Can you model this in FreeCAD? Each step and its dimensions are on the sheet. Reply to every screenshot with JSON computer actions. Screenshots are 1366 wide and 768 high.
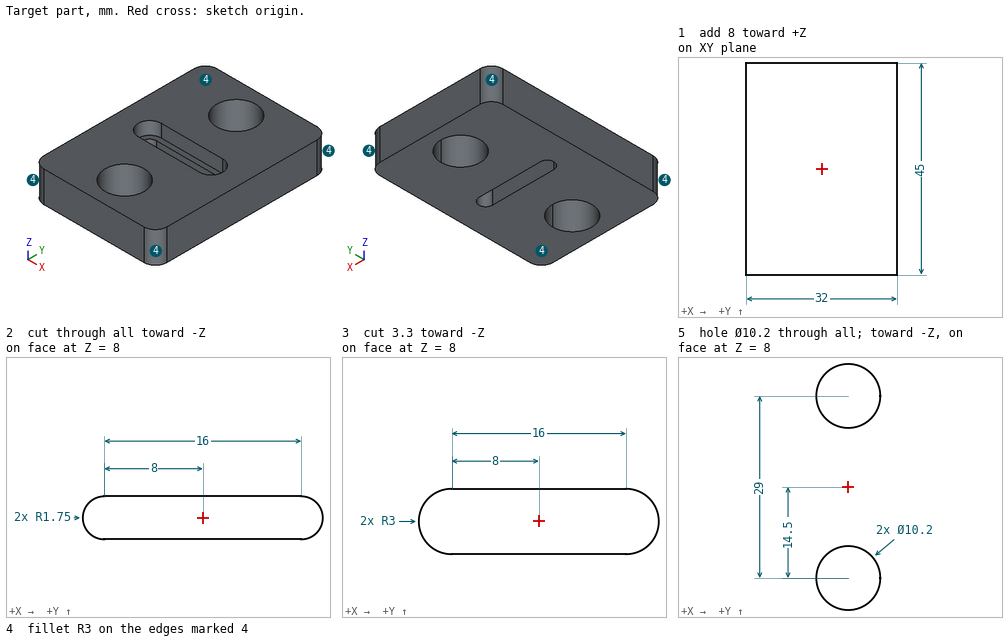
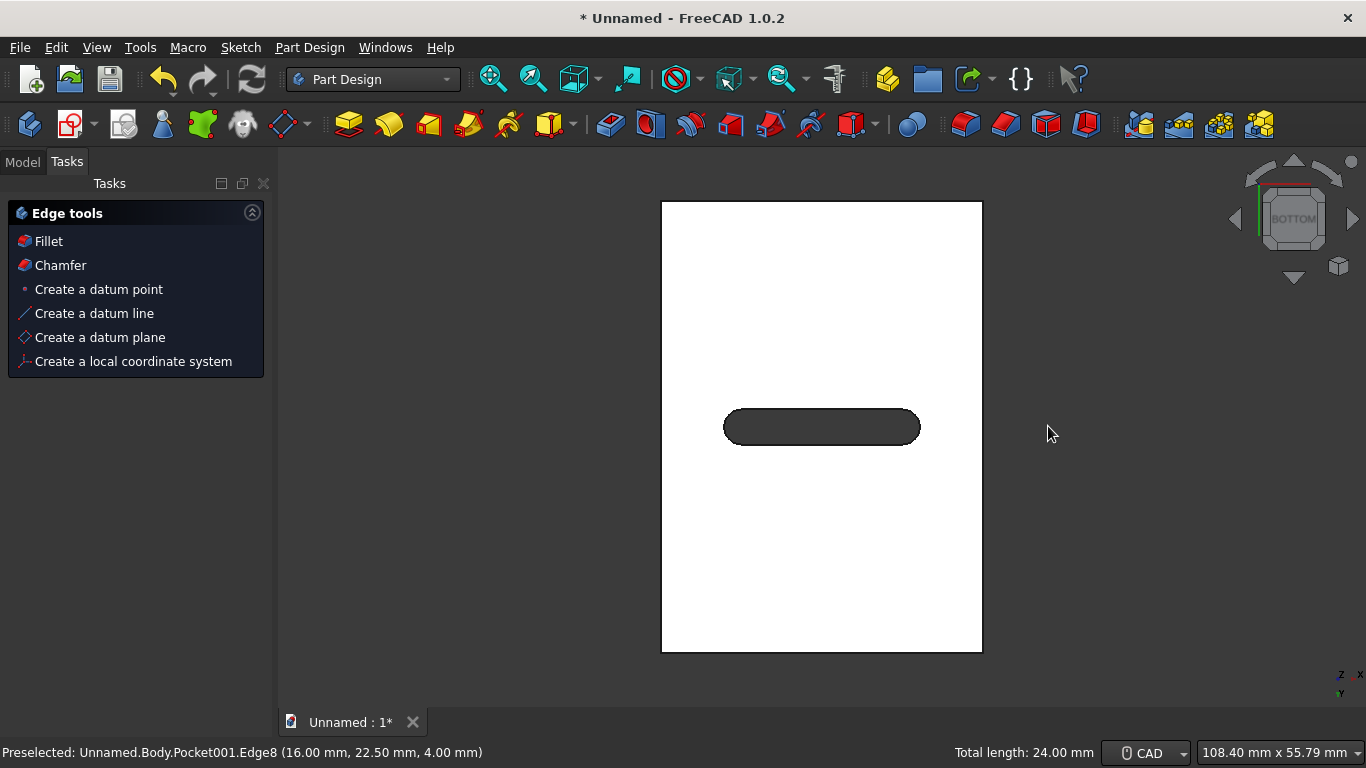
{"action": "key", "text": "4"}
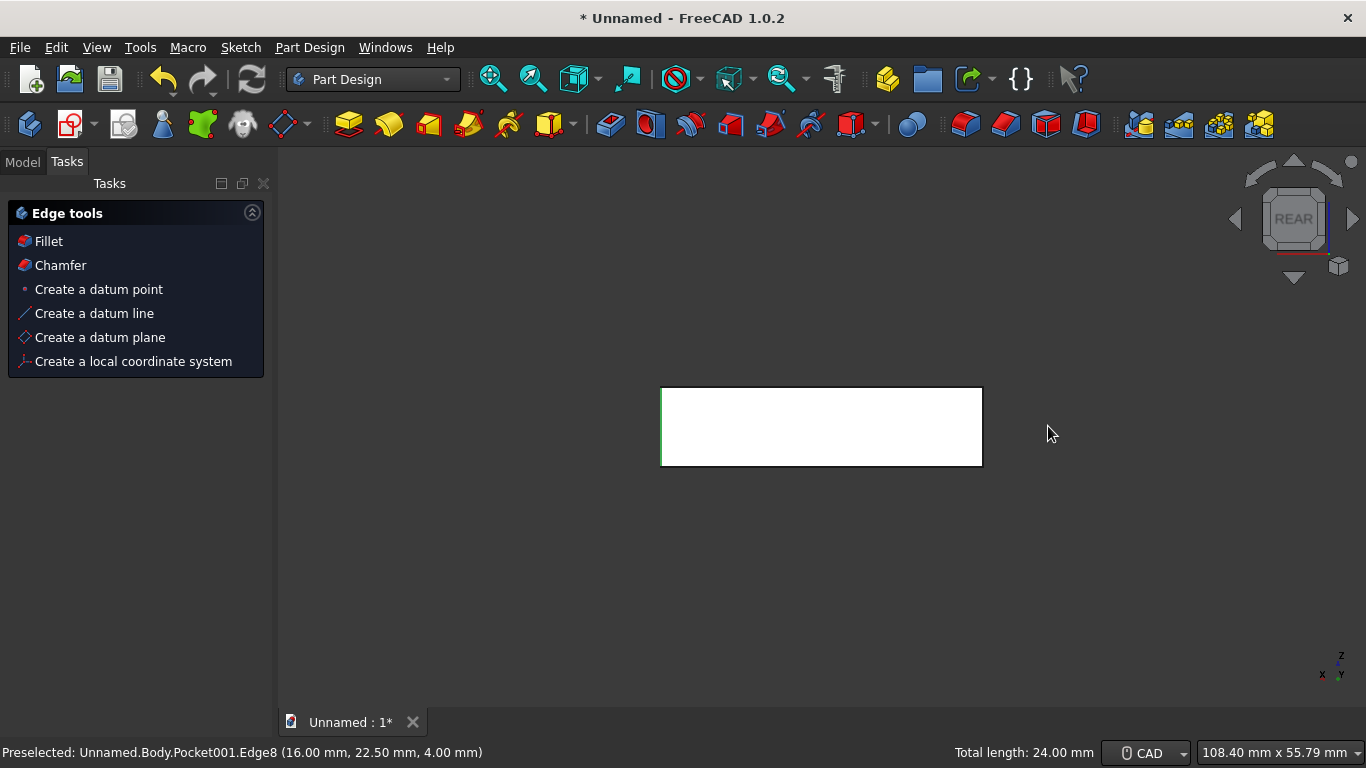
{"action": "key", "text": "v f"}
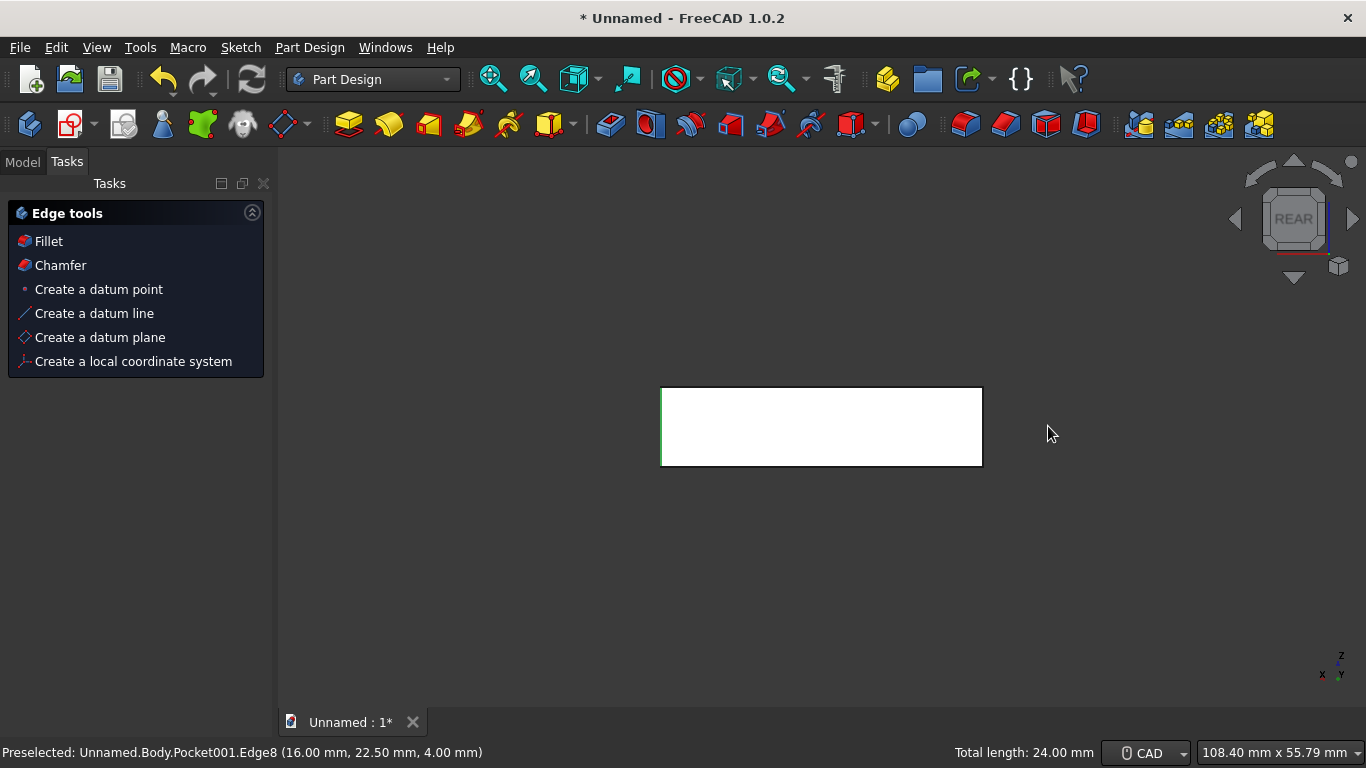
{"action": "left_click", "coordinate": [983, 426], "text": "ctrl"}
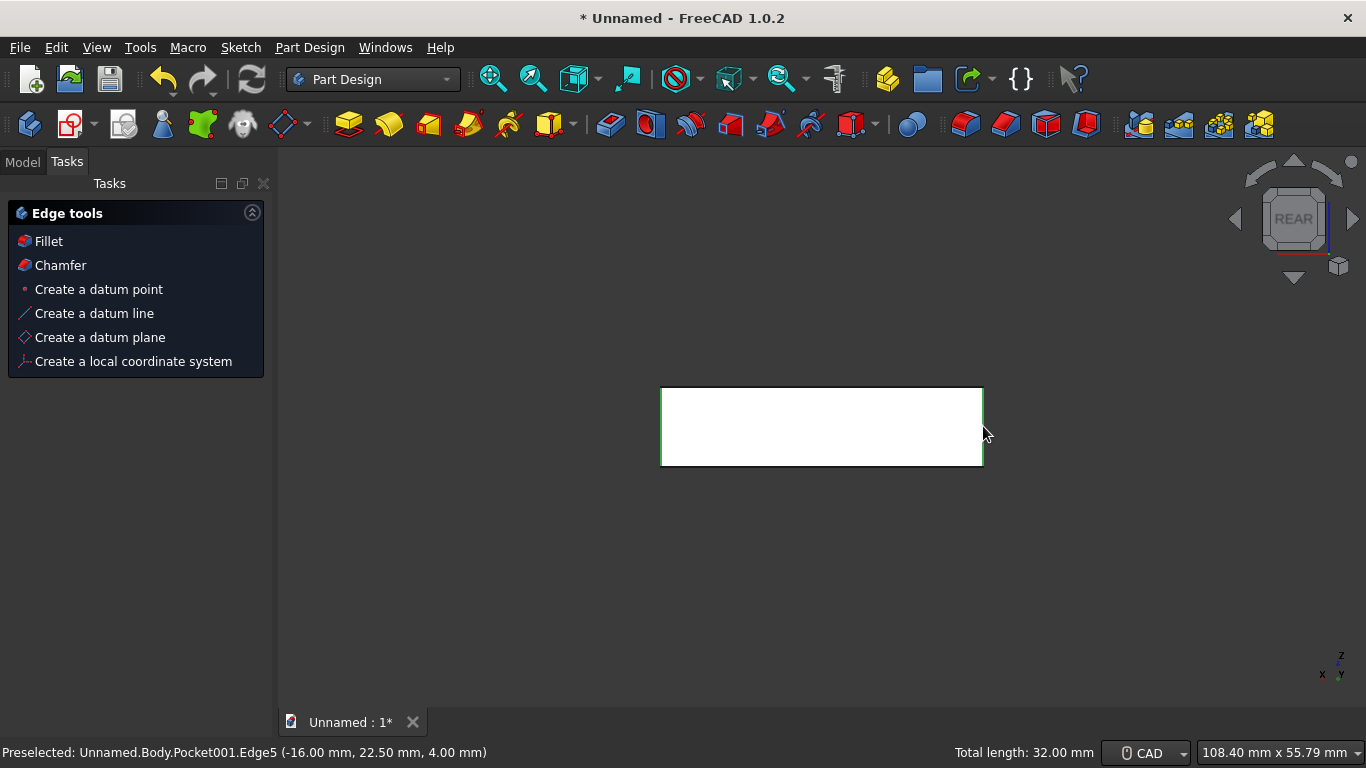
{"action": "left_click", "coordinate": [966, 124]}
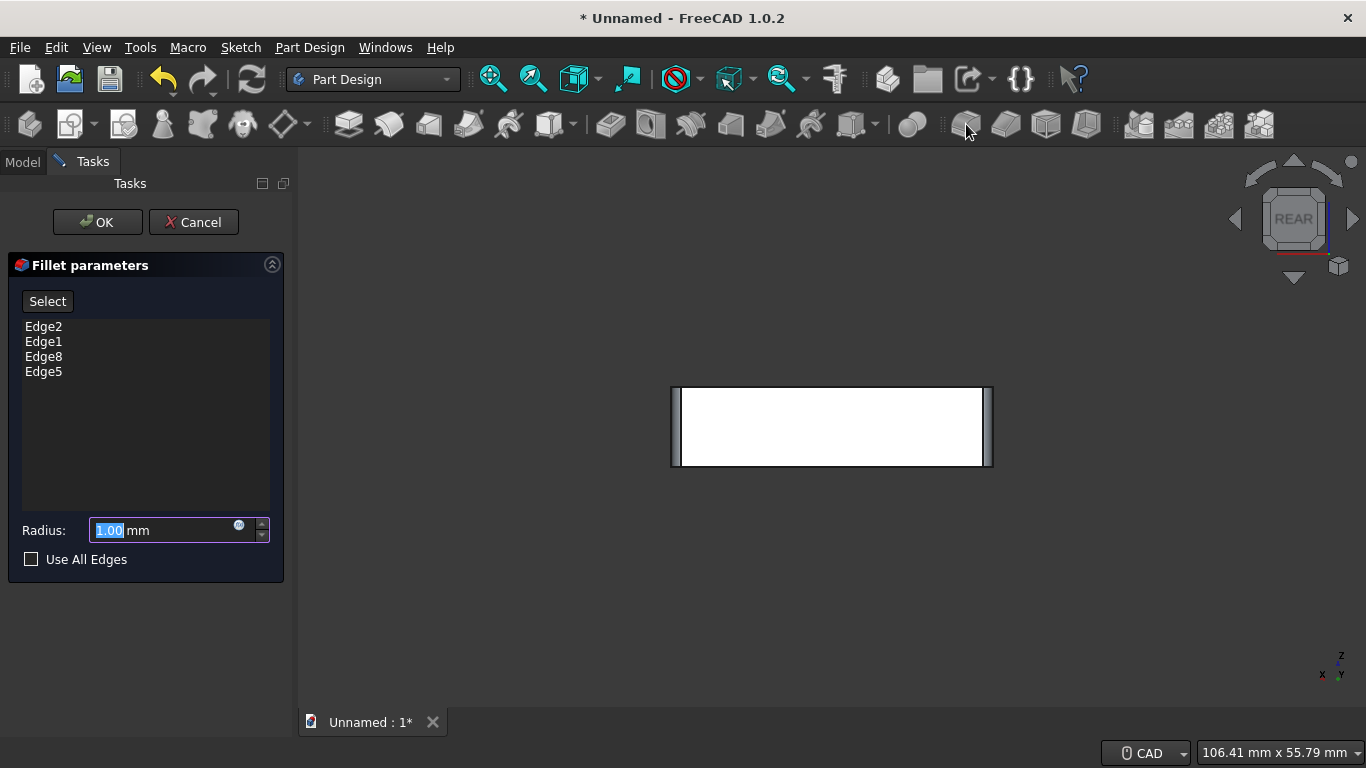
{"action": "type", "text": "3"}
{"action": "key", "text": "Tab"}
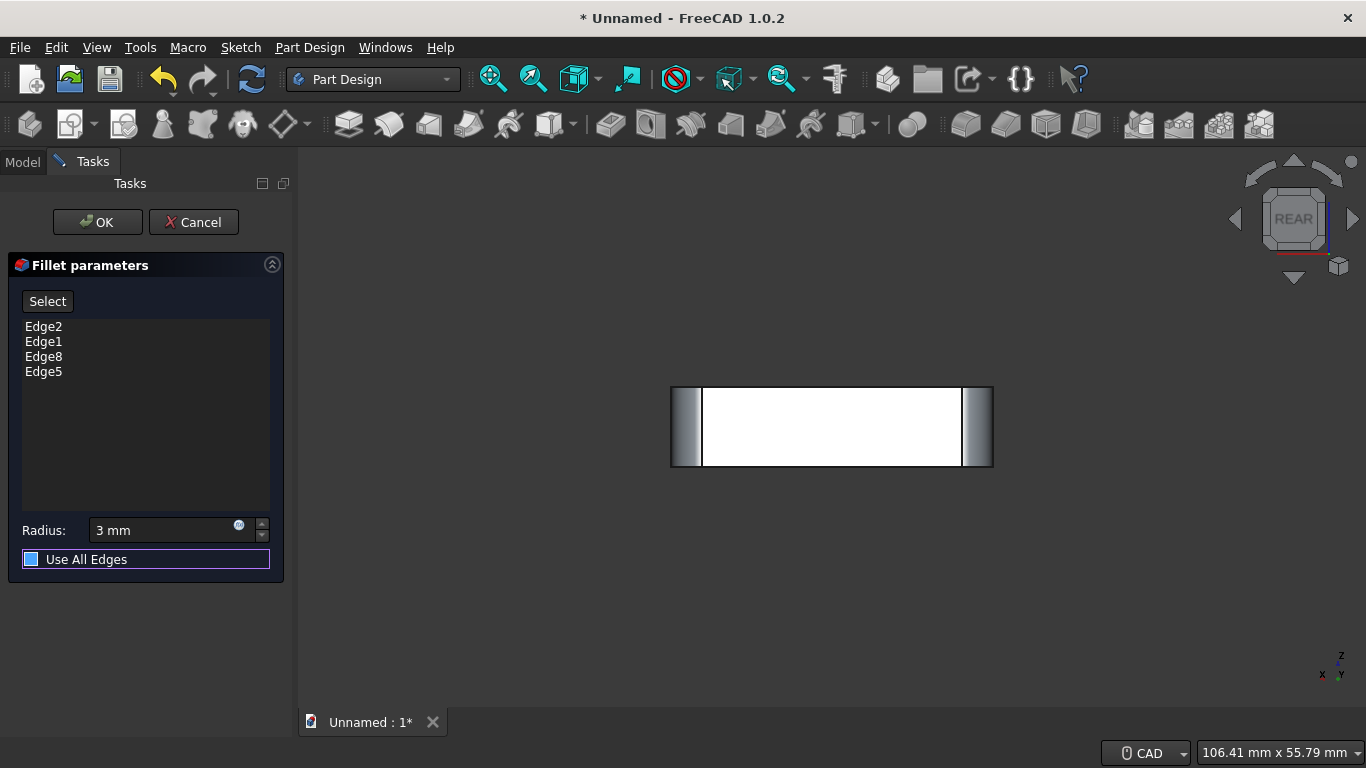
{"action": "left_click", "coordinate": [98, 222]}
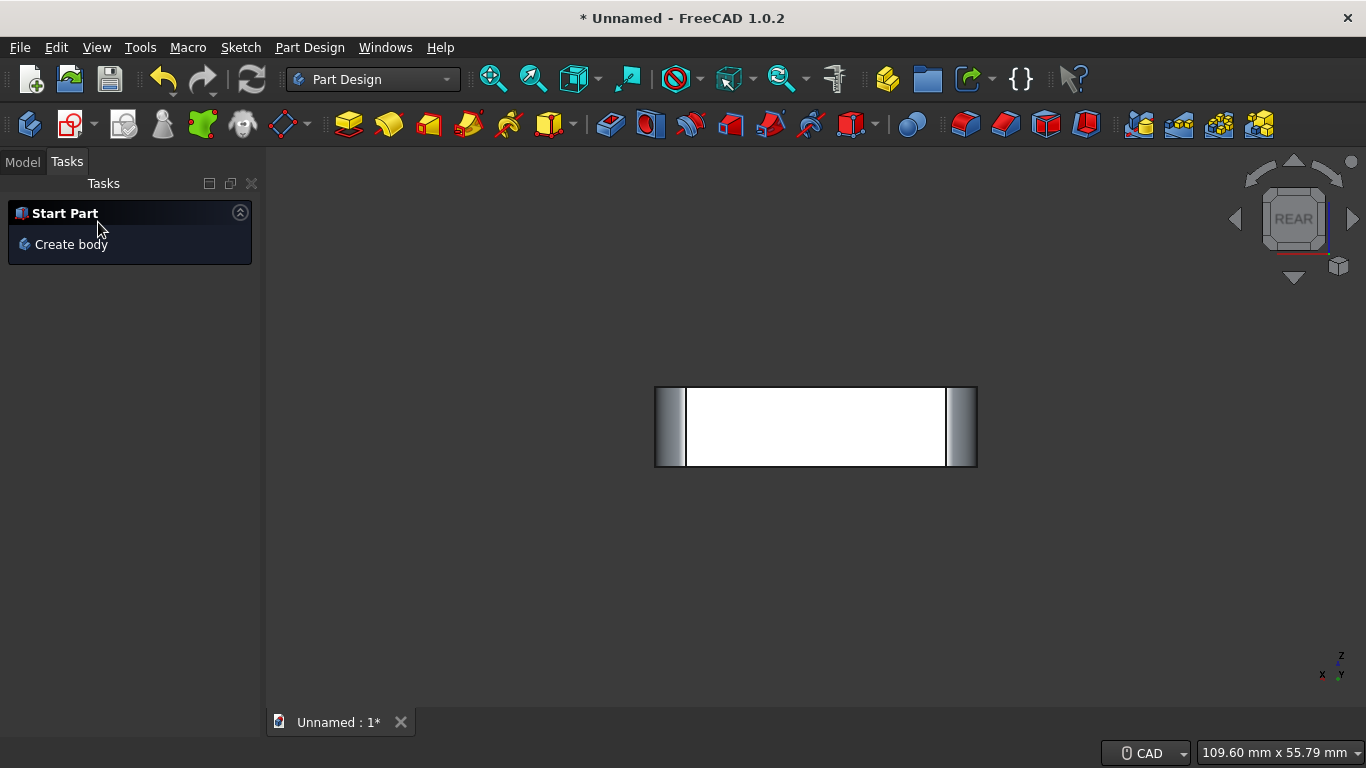
{"action": "left_click", "coordinate": [494, 80]}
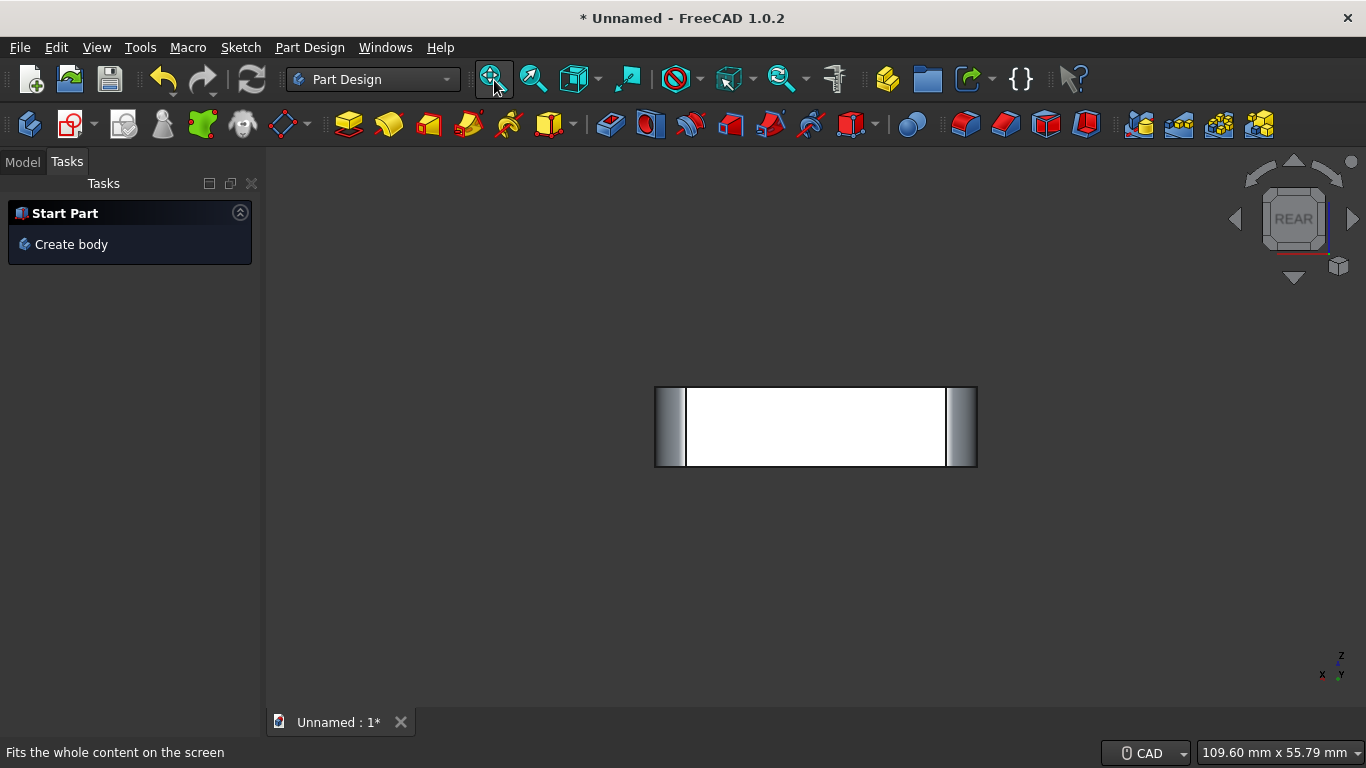
{"action": "key", "text": "0"}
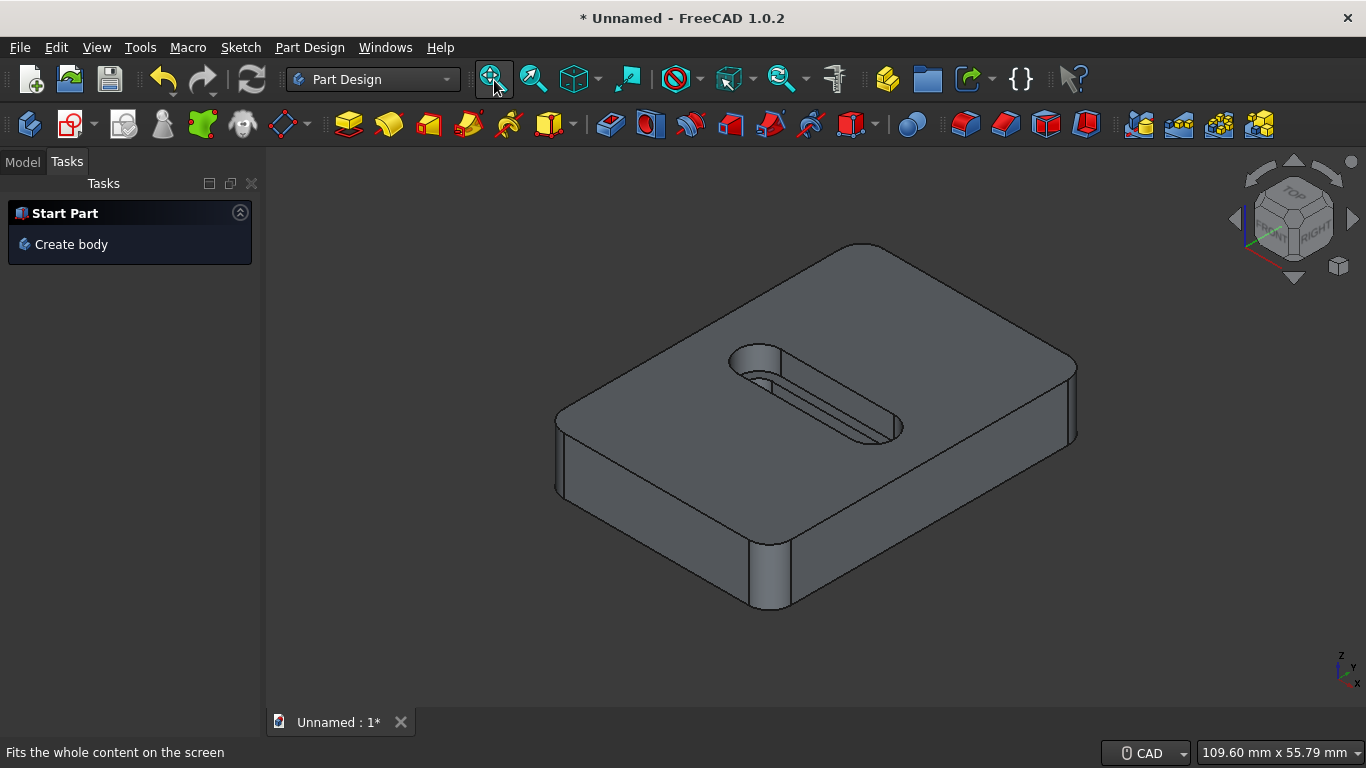
{"action": "left_click", "coordinate": [940, 359]}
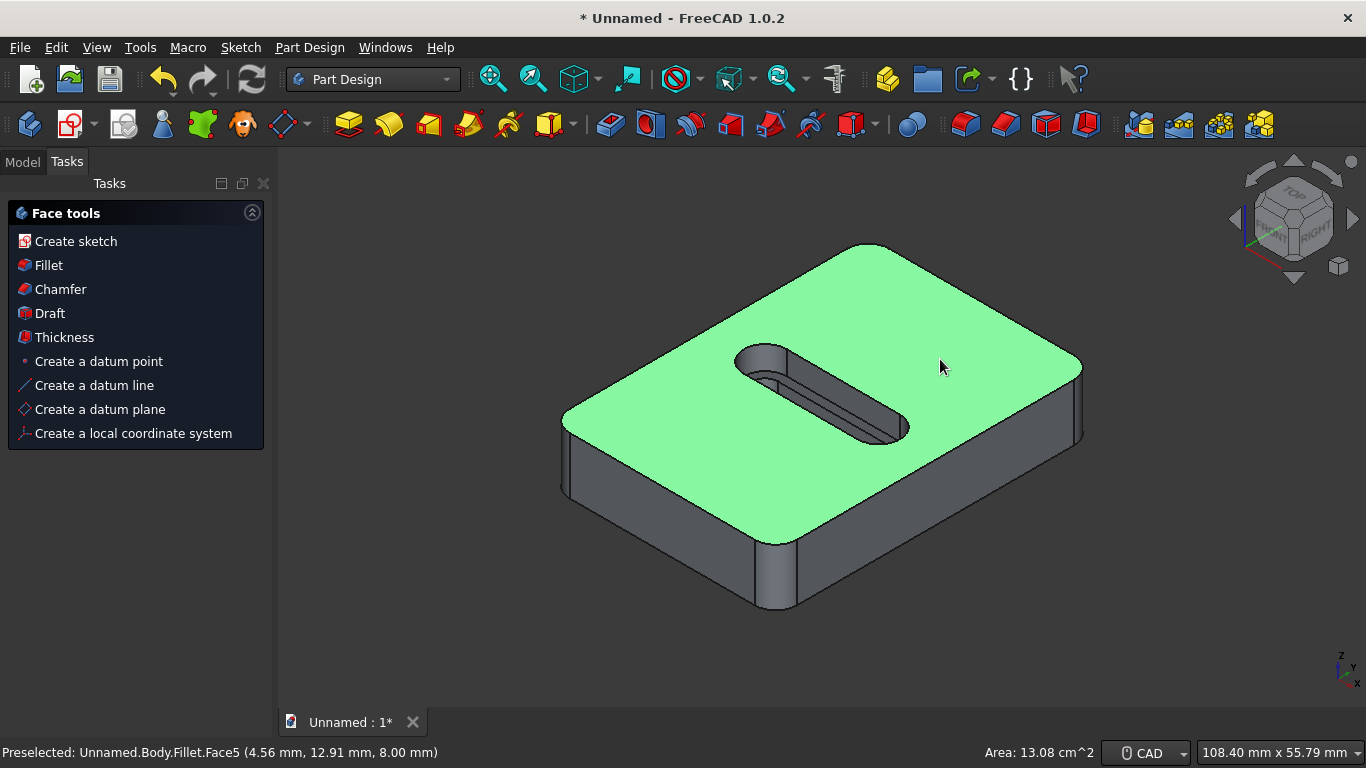
{"action": "left_click", "coordinate": [70, 124]}